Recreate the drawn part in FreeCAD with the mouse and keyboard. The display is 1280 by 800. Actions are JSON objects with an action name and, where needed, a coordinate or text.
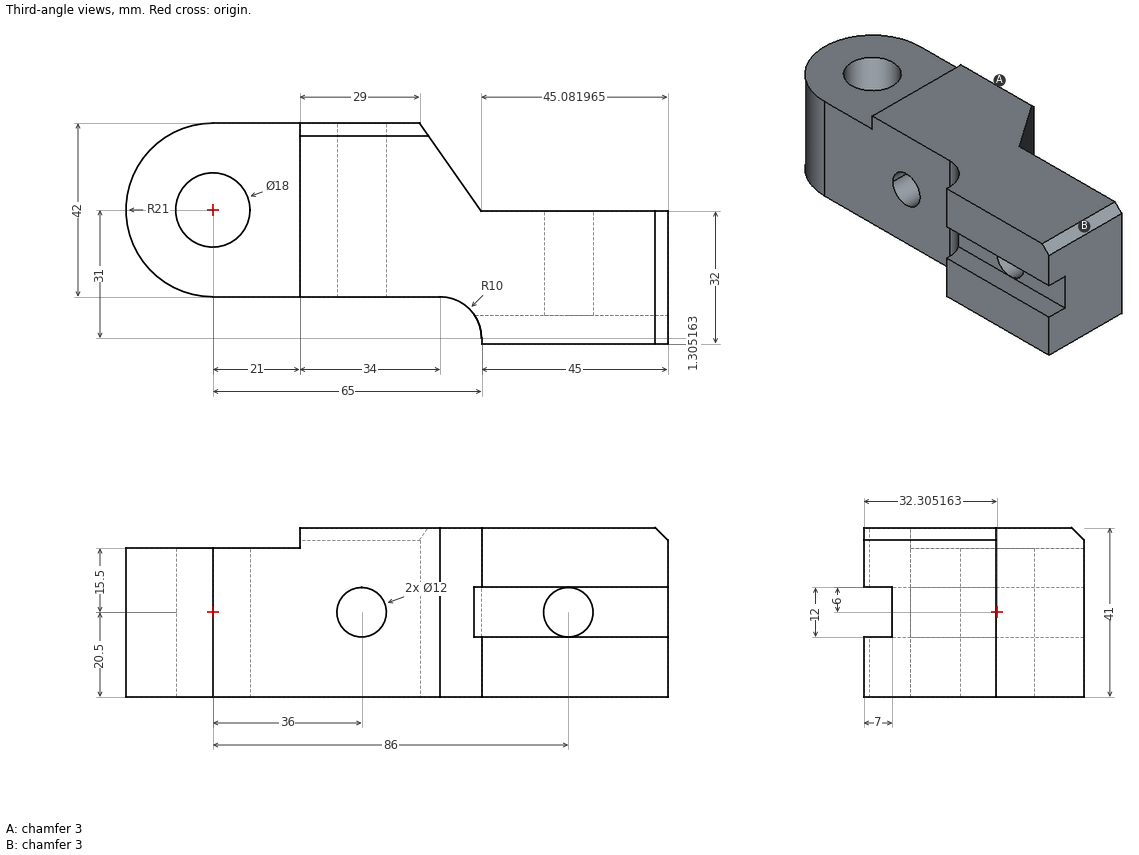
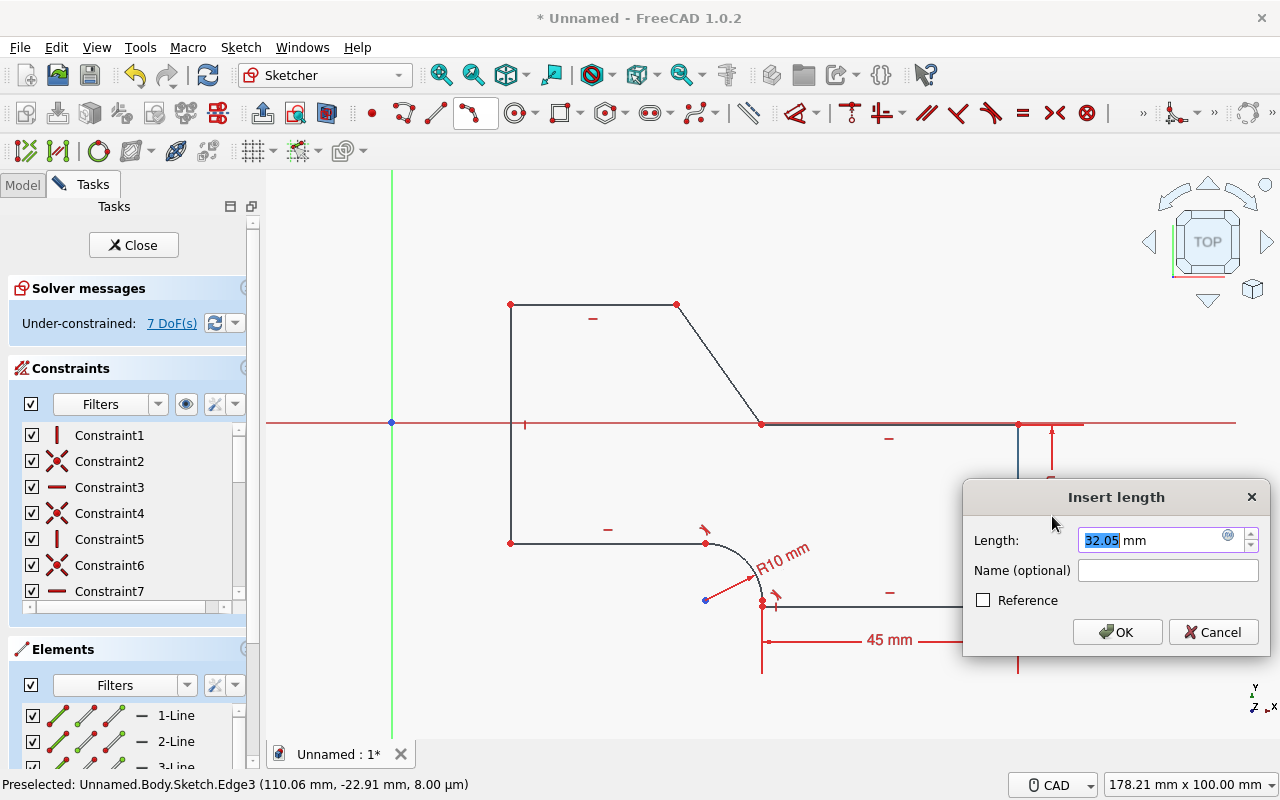
{"action": "type", "text": "32"}
{"action": "key", "text": "Return"}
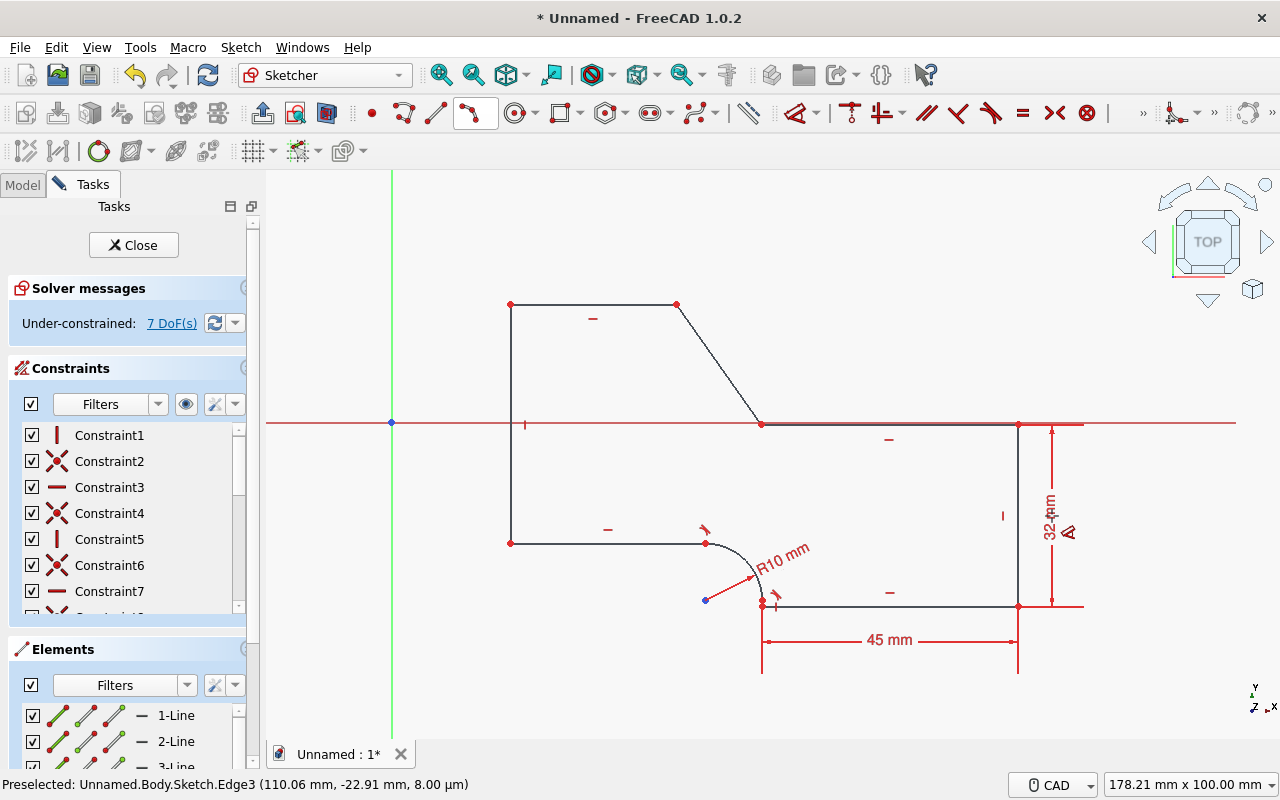
{"action": "left_click", "coordinate": [627, 305]}
{"action": "left_click", "coordinate": [594, 271]}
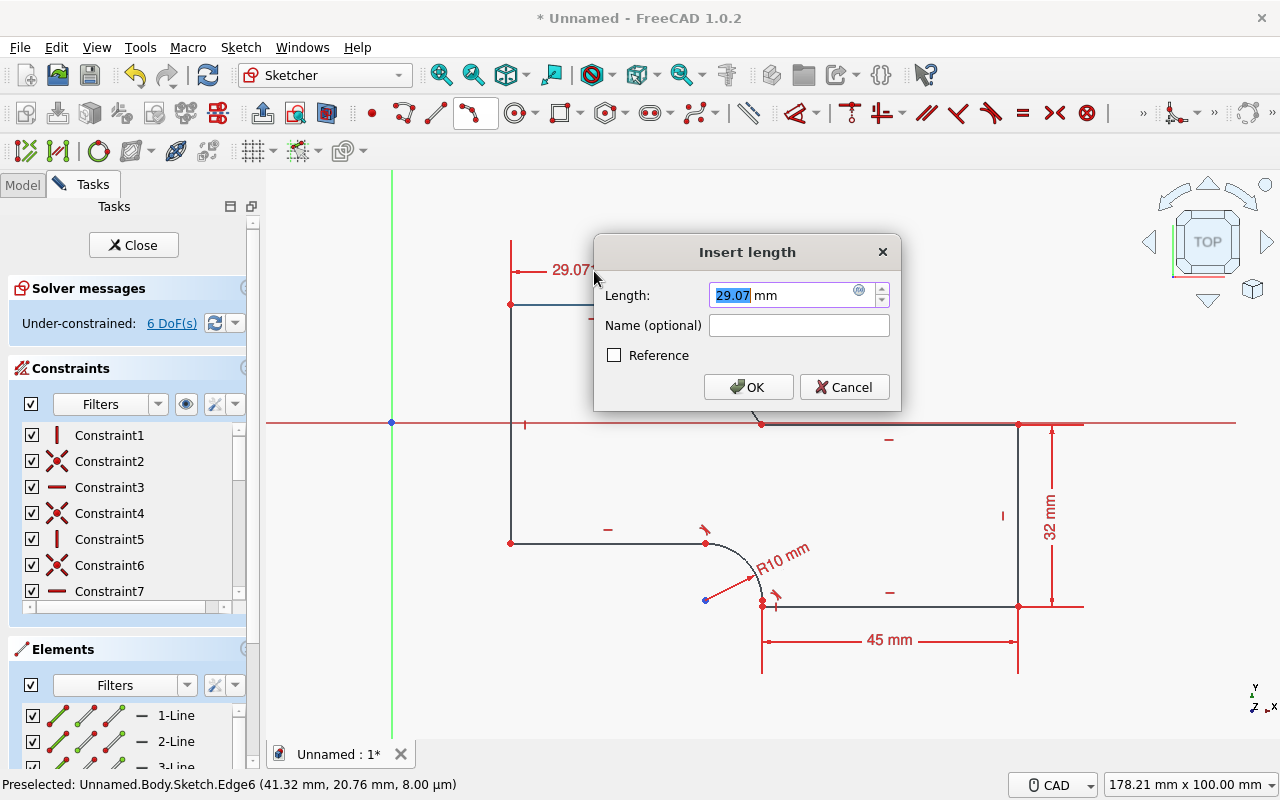
{"action": "type", "text": "29"}
{"action": "key", "text": "Return"}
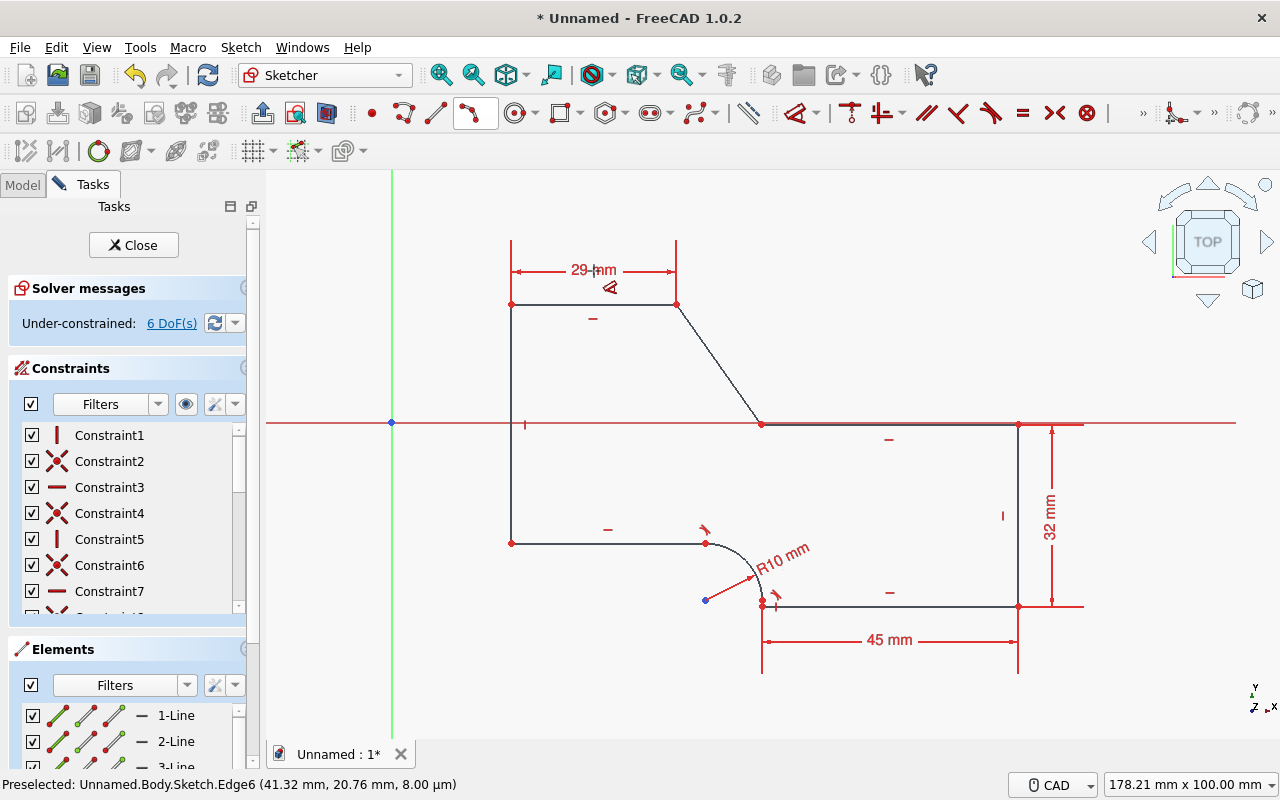
{"action": "left_click", "coordinate": [511, 376]}
{"action": "left_click", "coordinate": [477, 369]}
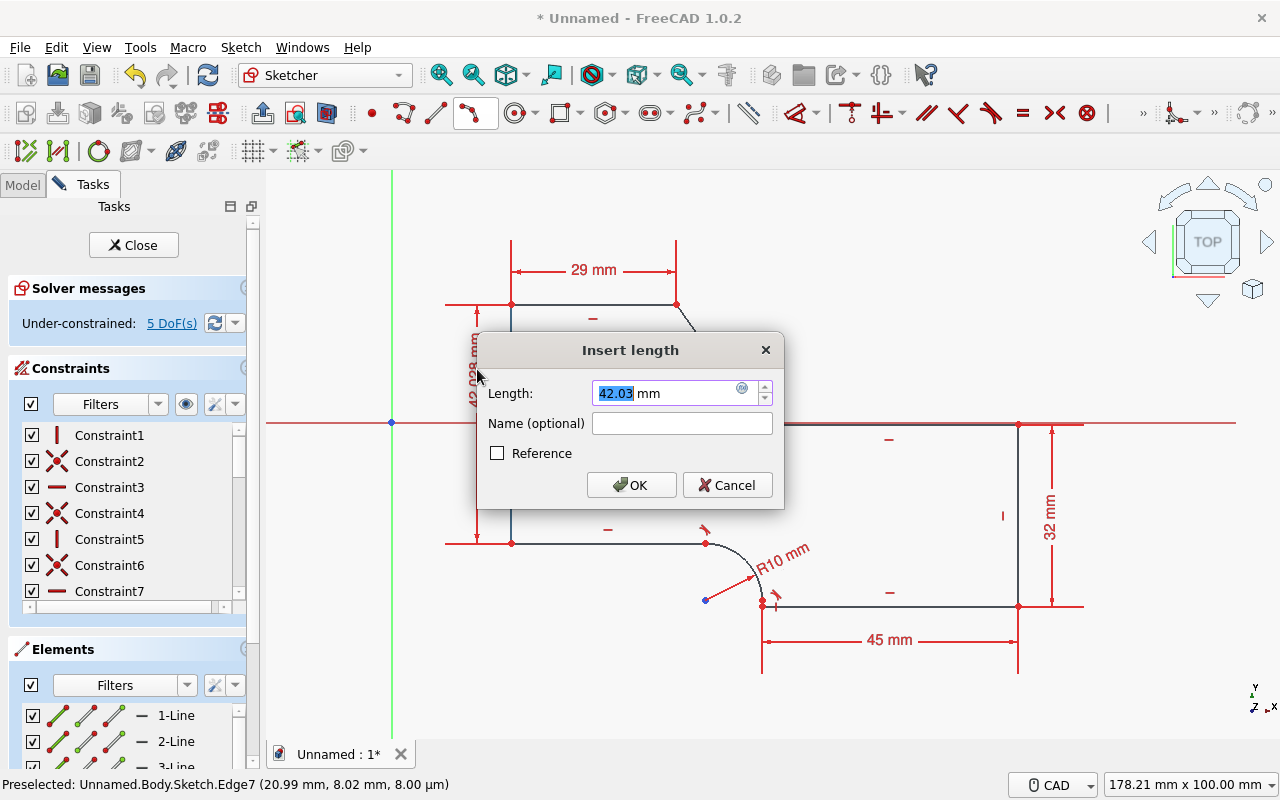
{"action": "type", "text": "42"}
{"action": "key", "text": "Return"}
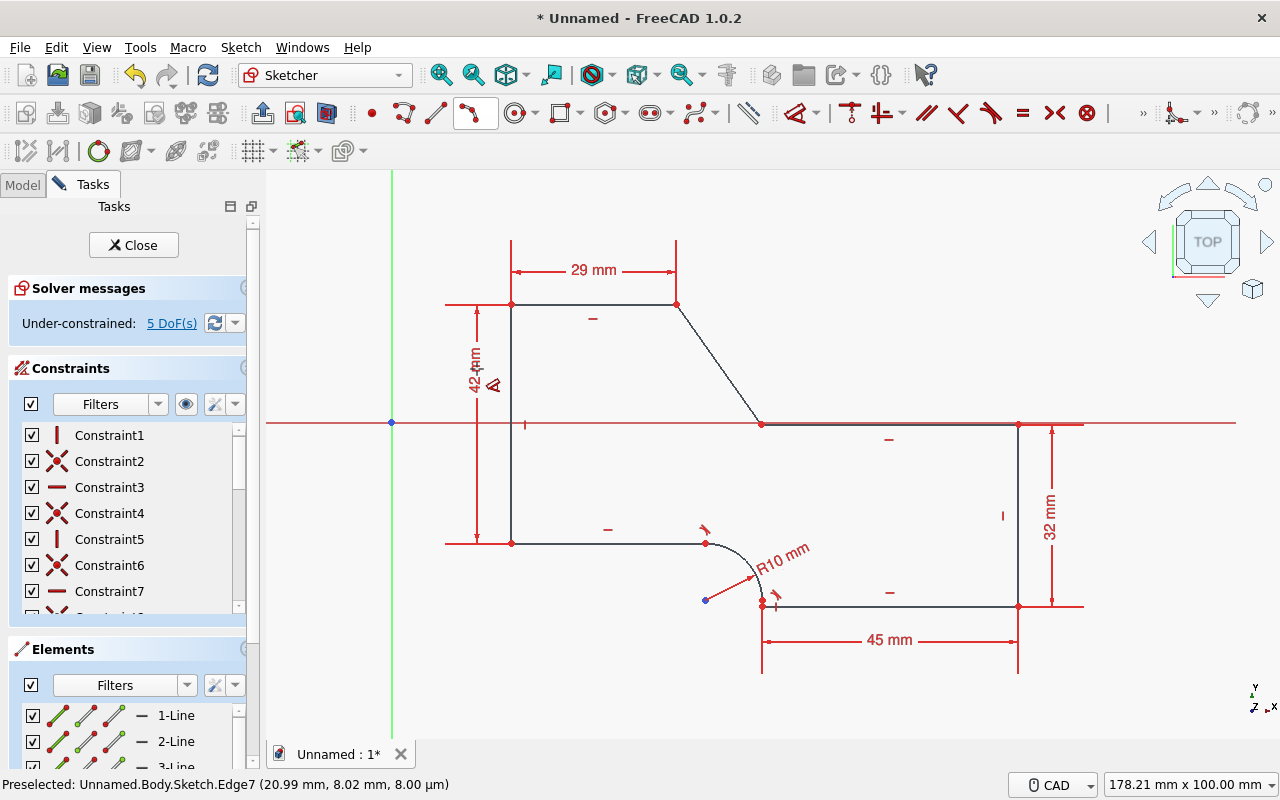
{"action": "left_click", "coordinate": [569, 544]}
{"action": "left_click", "coordinate": [608, 578]}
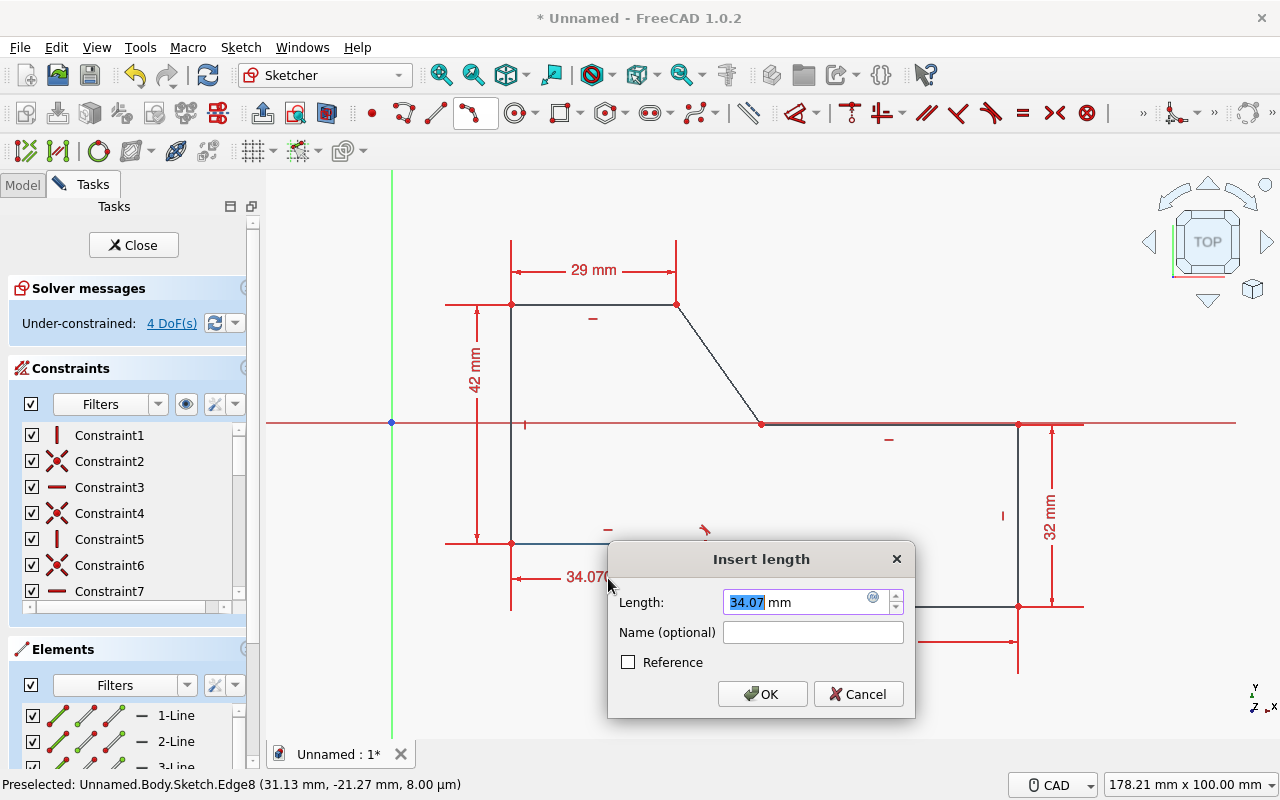
{"action": "type", "text": "34"}
{"action": "key", "text": "Return"}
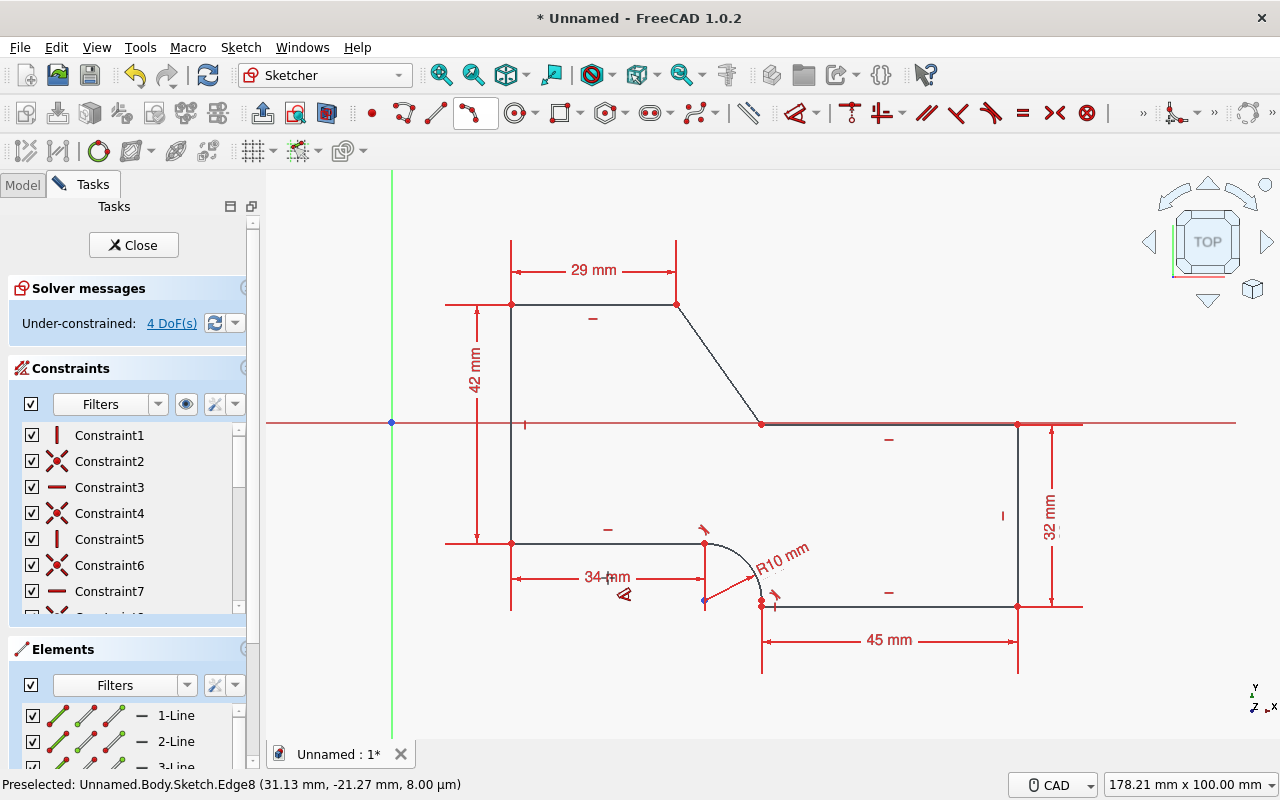
{"action": "scroll", "coordinate": [762, 601], "scroll_direction": "up", "scroll_amount": 4}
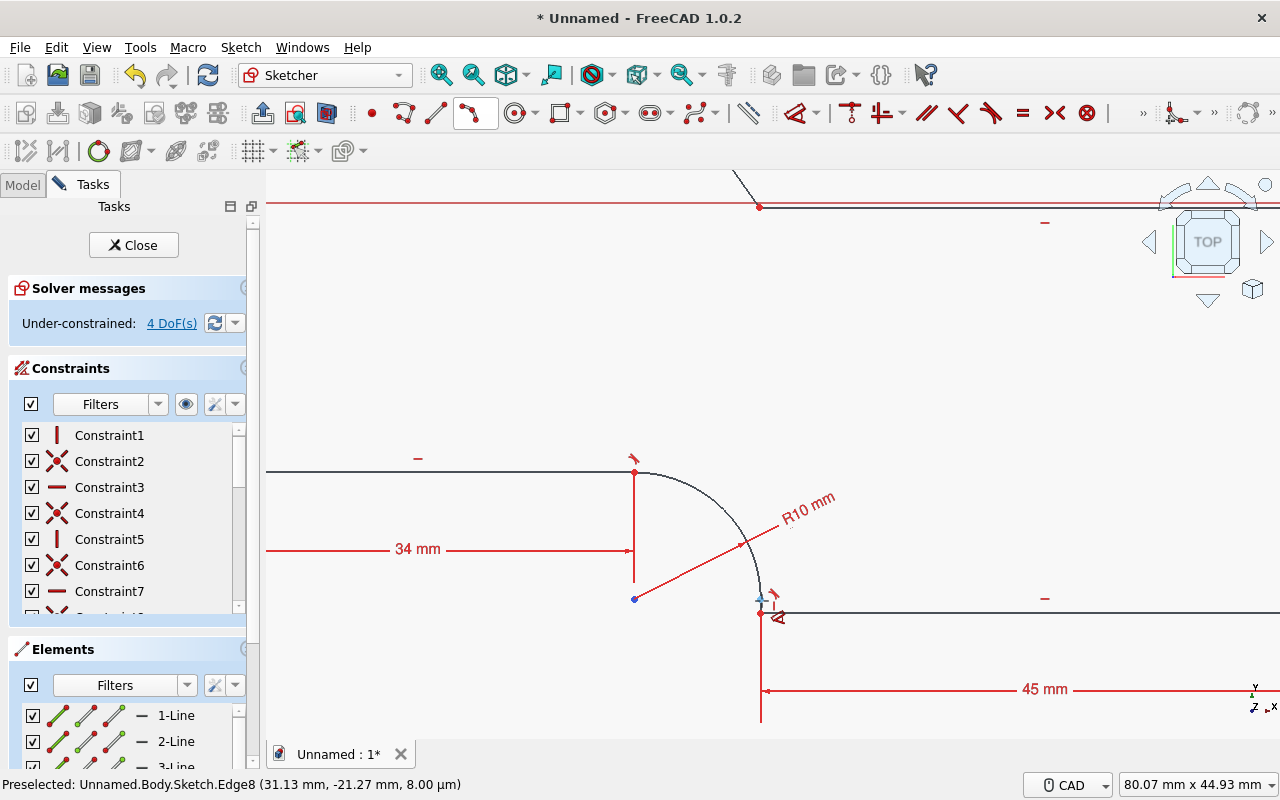
{"action": "left_click", "coordinate": [761, 599]}
{"action": "left_click", "coordinate": [527, 633]}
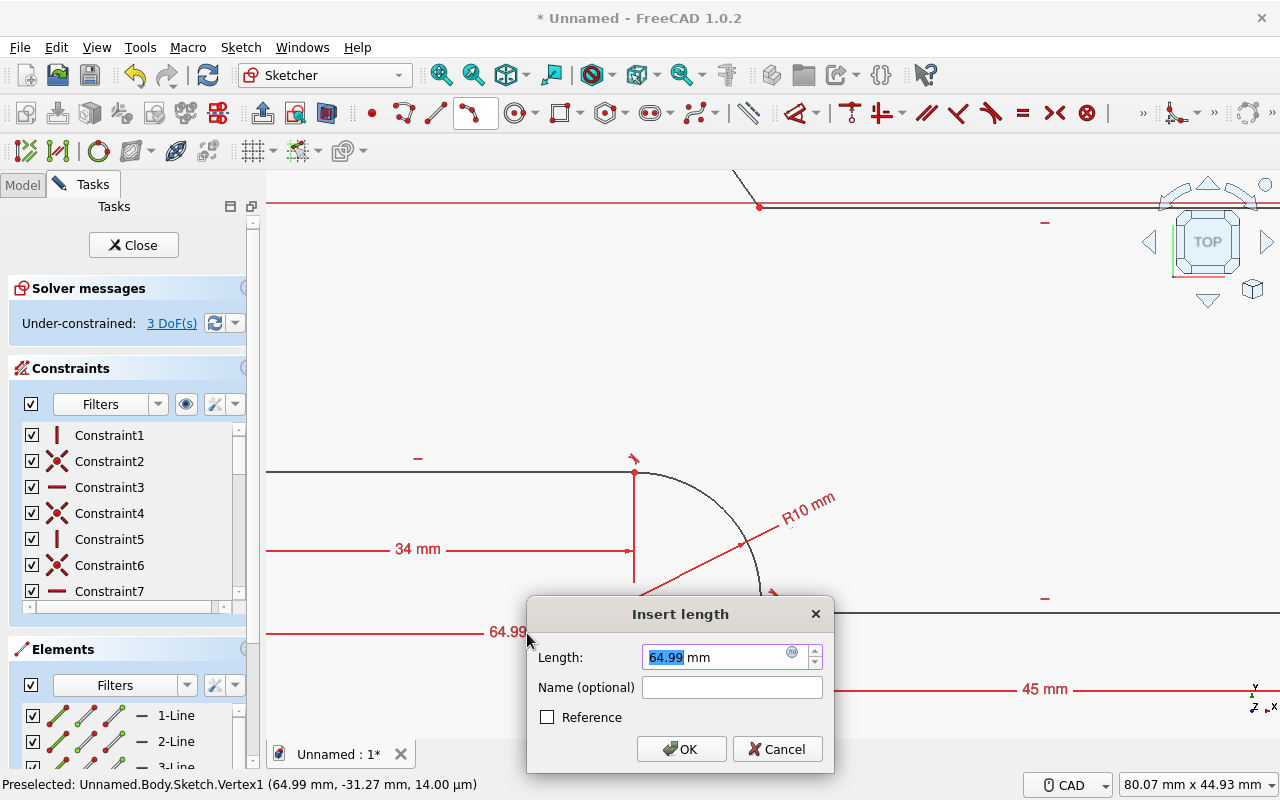
{"action": "type", "text": "65"}
{"action": "key", "text": "Return"}